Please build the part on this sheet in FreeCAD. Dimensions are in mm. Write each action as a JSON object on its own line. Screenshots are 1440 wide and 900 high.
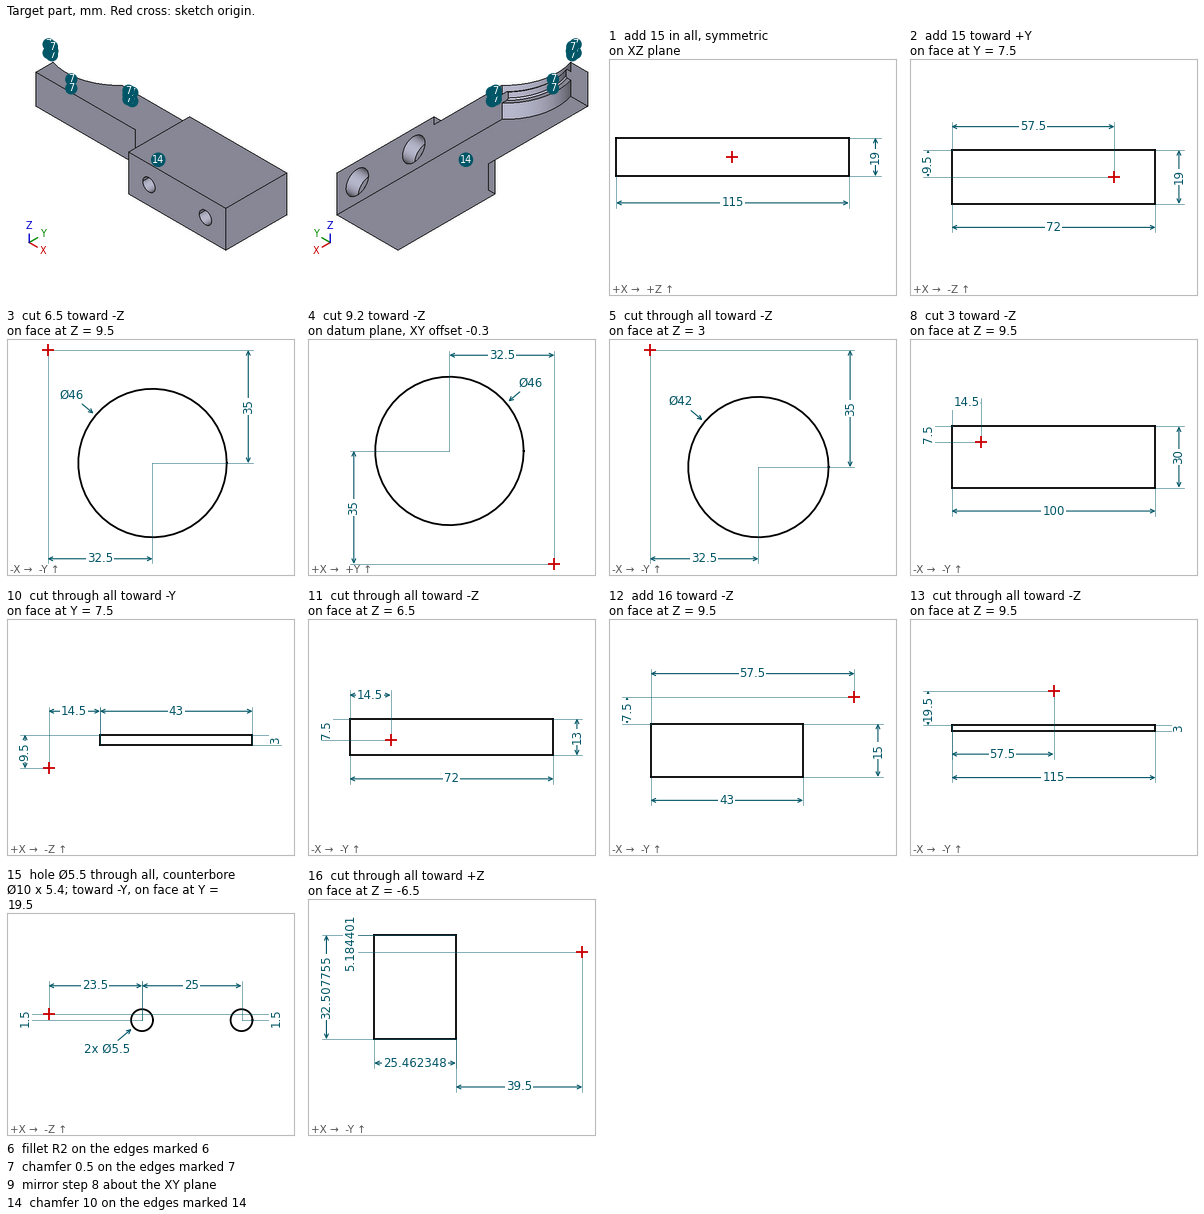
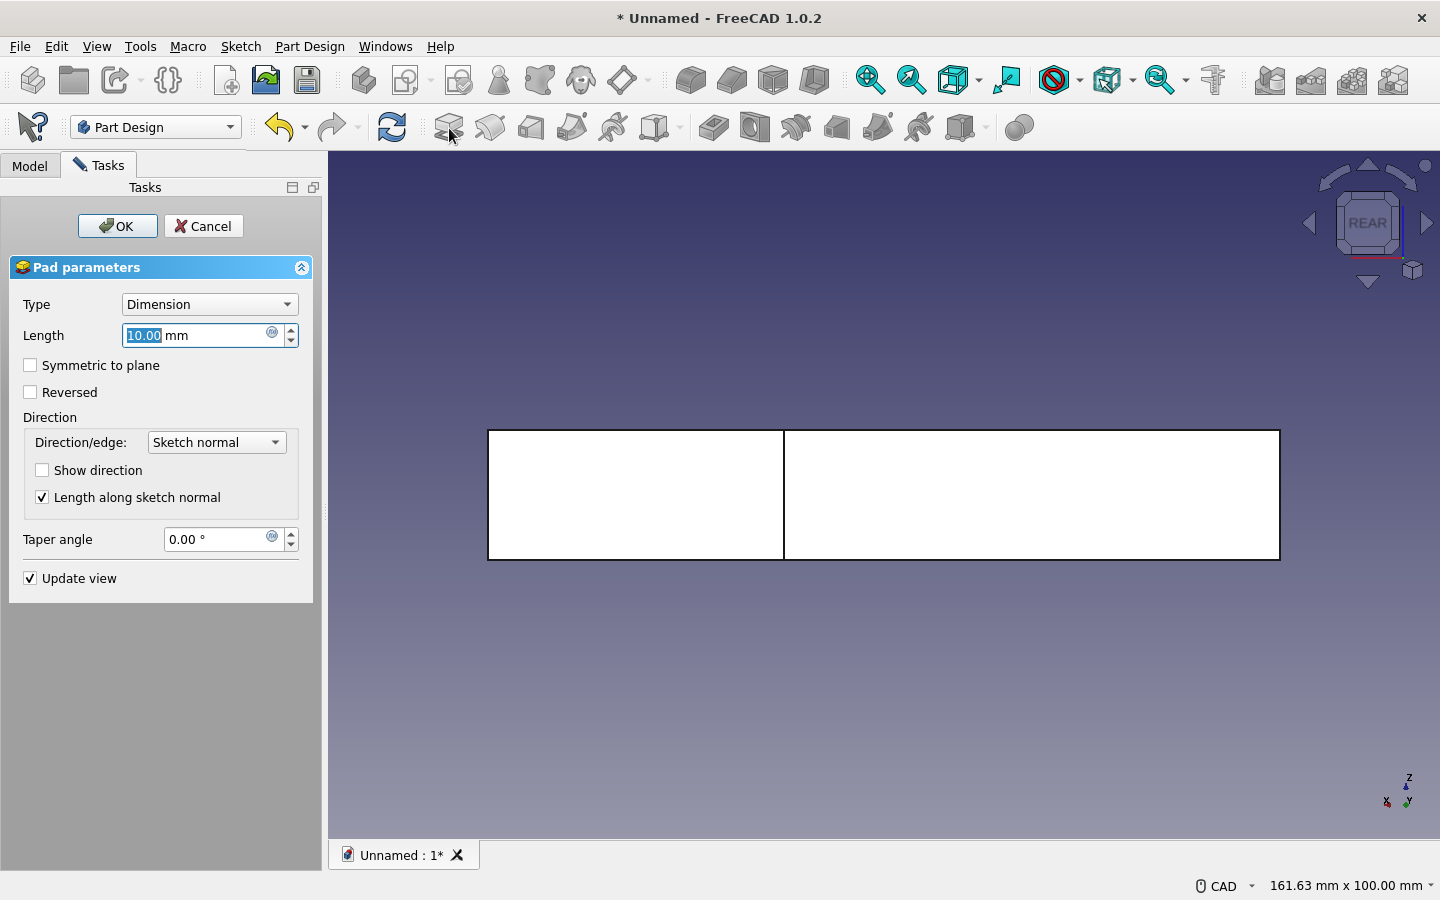
{"action": "type", "text": "15"}
{"action": "key", "text": "Tab"}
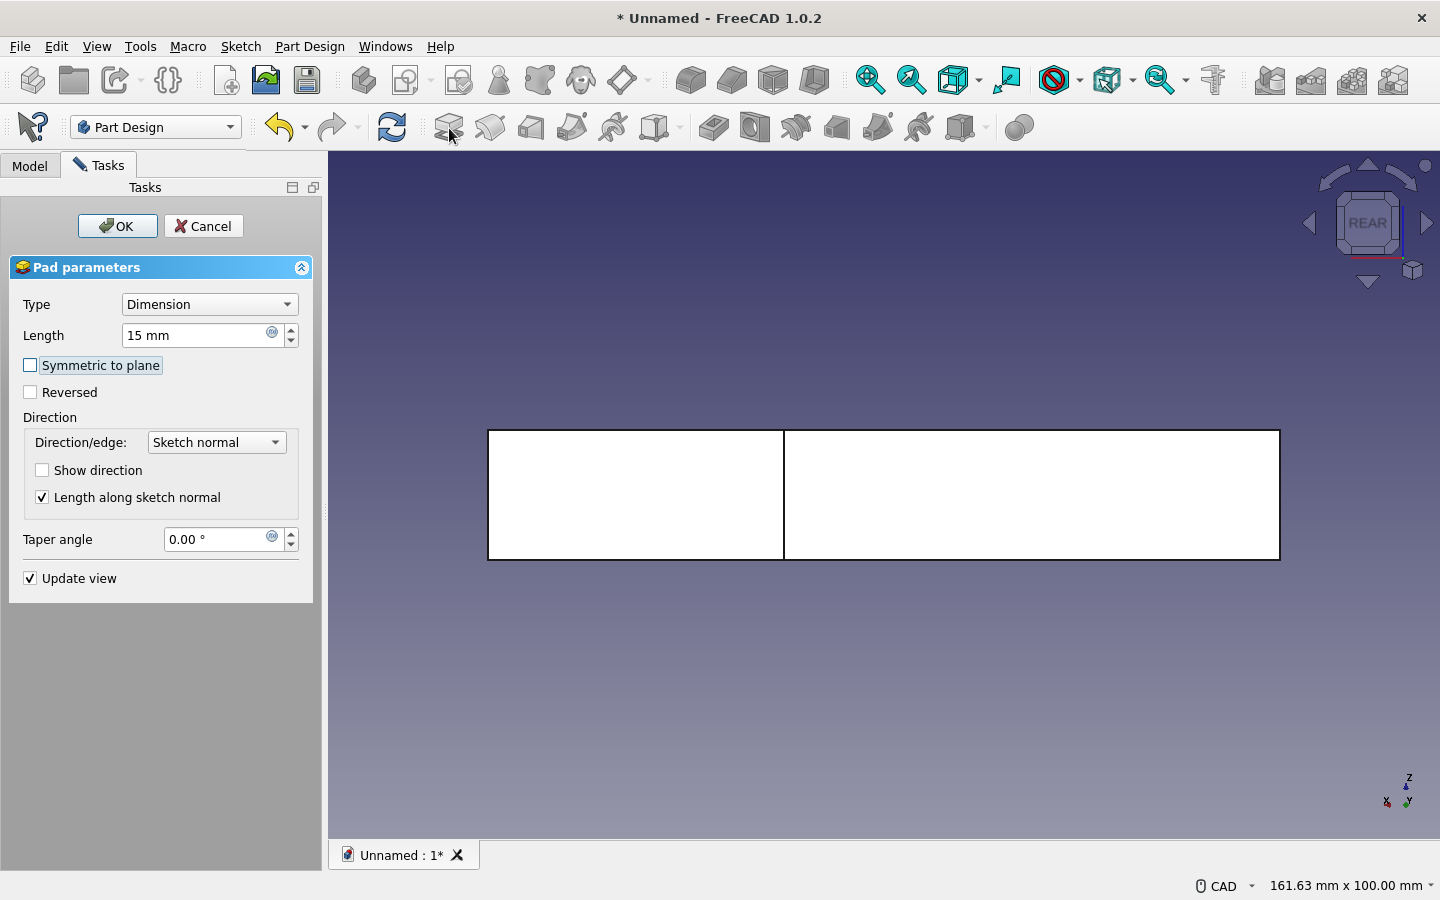
{"action": "left_click", "coordinate": [118, 226]}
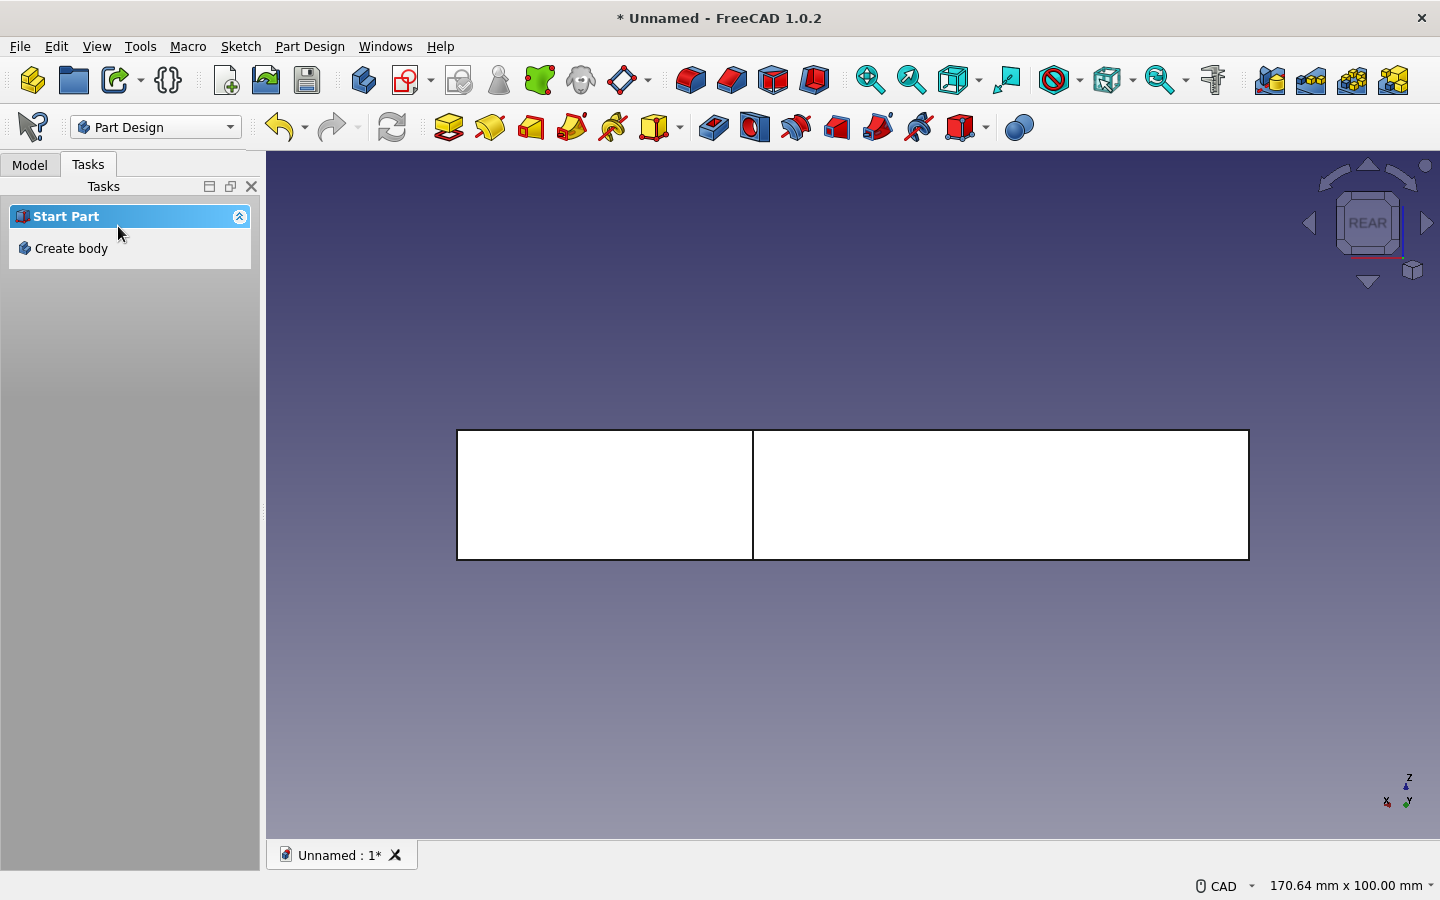
{"action": "key", "text": "0"}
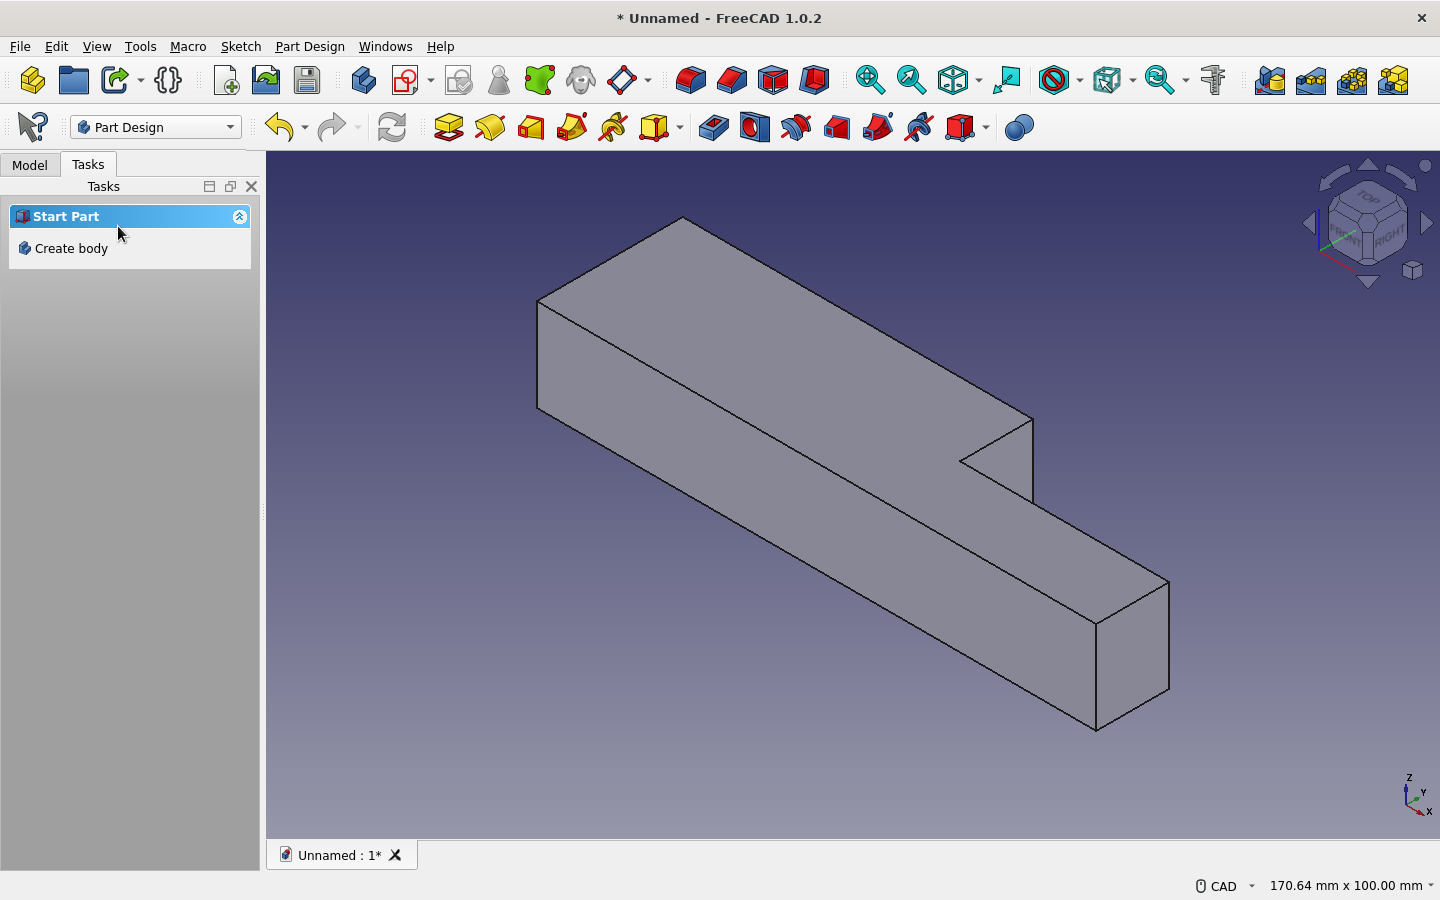
{"action": "left_click", "coordinate": [810, 373]}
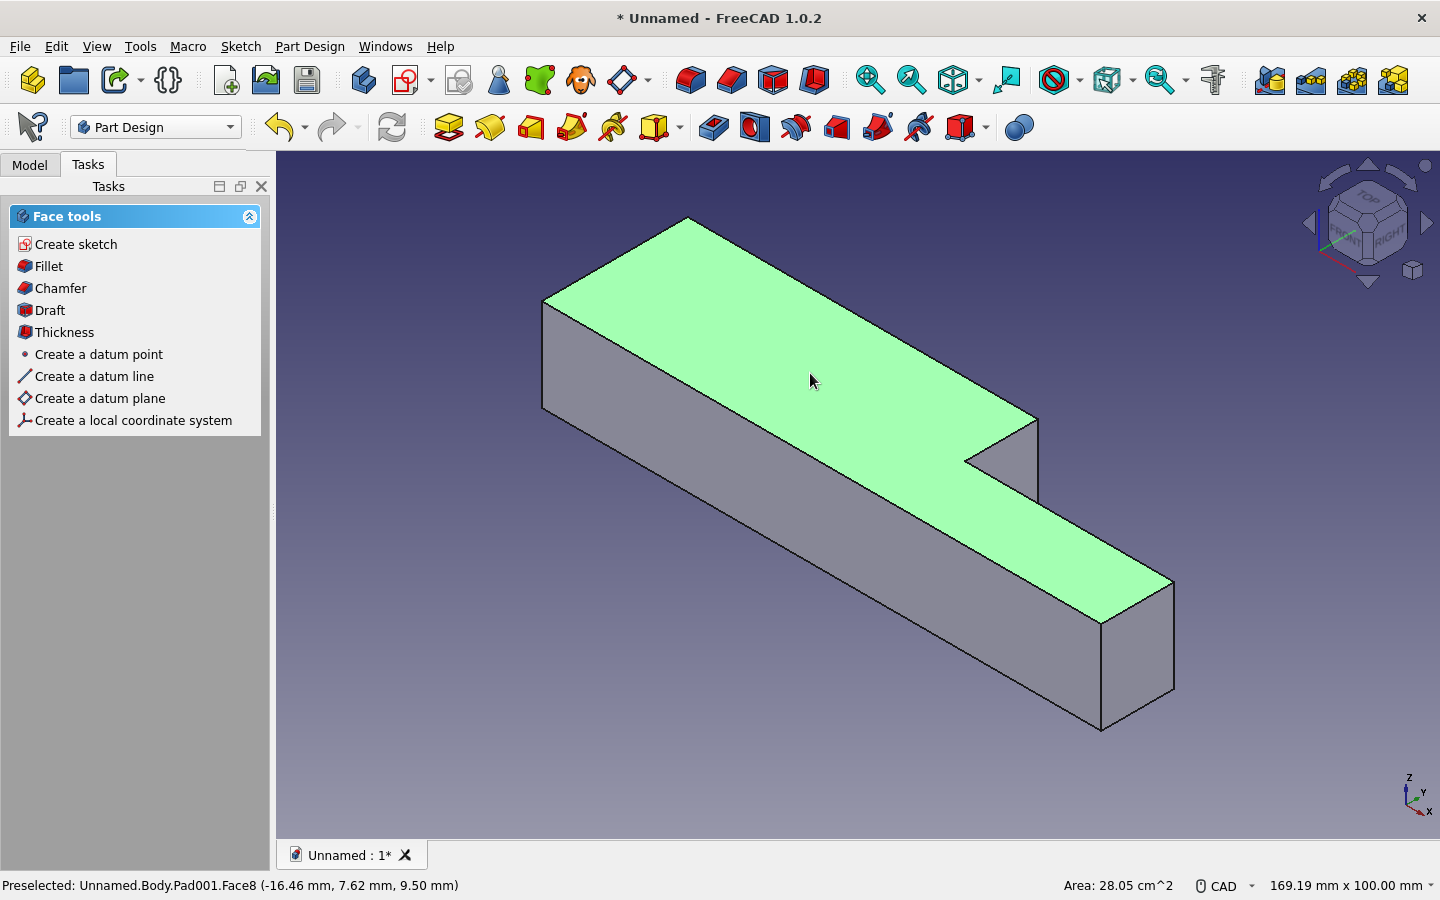
{"action": "left_click", "coordinate": [404, 80]}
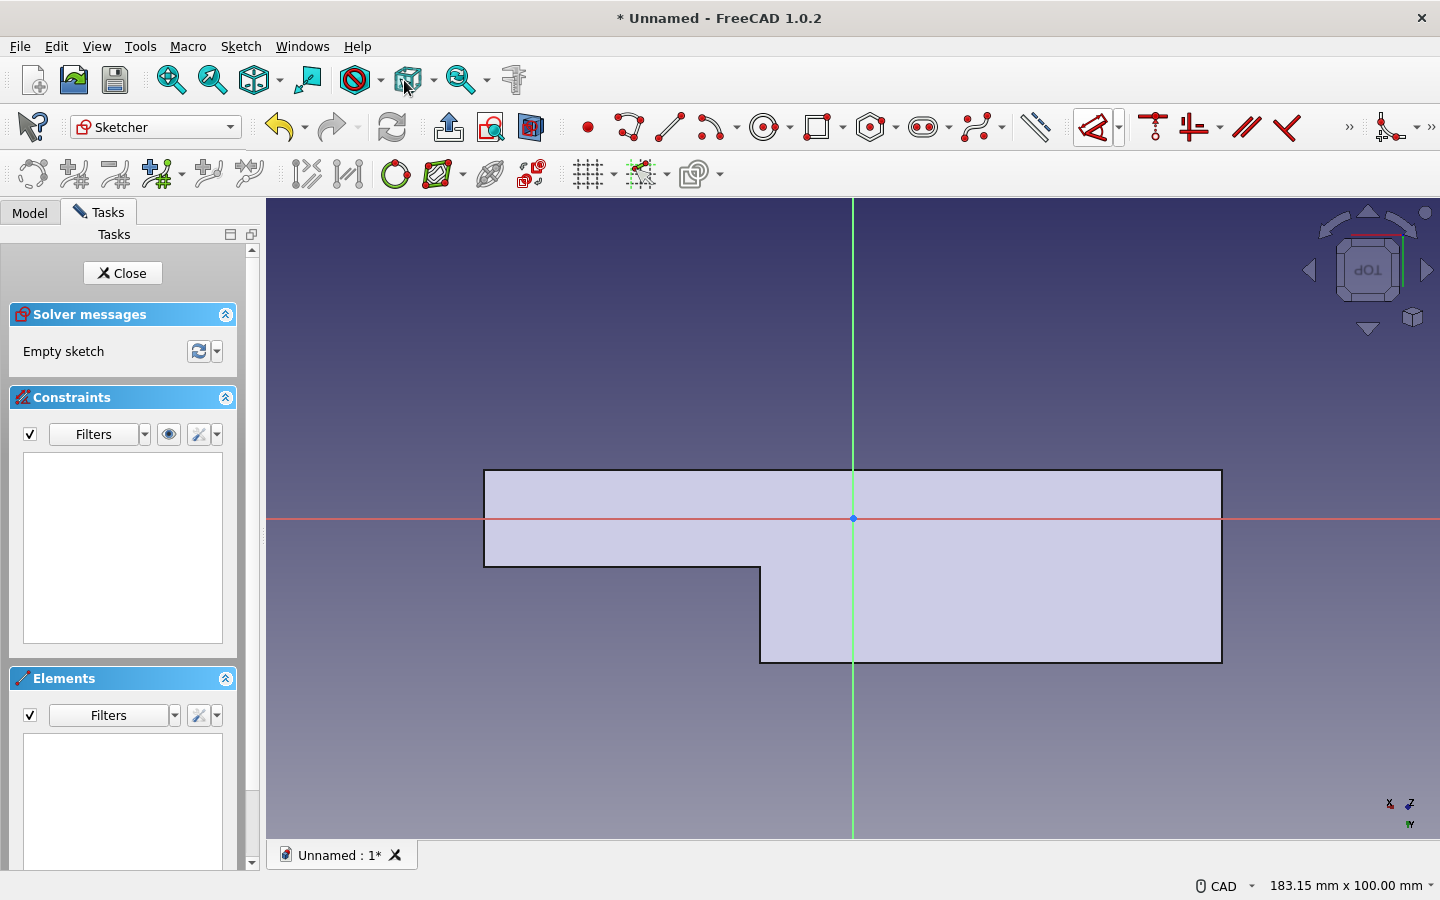
{"action": "scroll", "coordinate": [294, 226], "scroll_direction": "down", "scroll_amount": 1}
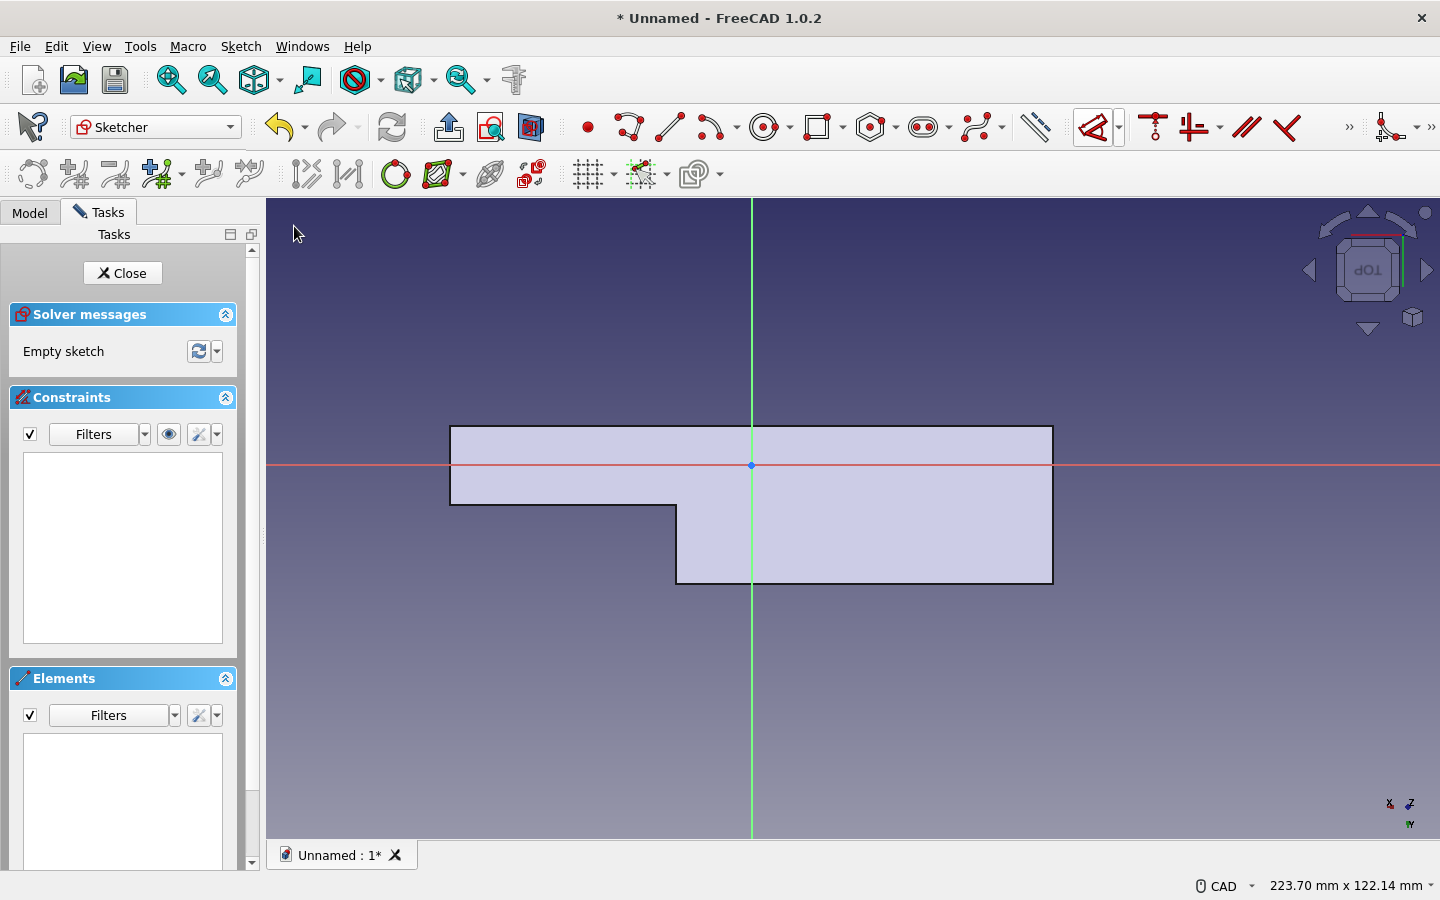
{"action": "scroll", "coordinate": [1127, 811], "scroll_direction": "up", "scroll_amount": 2}